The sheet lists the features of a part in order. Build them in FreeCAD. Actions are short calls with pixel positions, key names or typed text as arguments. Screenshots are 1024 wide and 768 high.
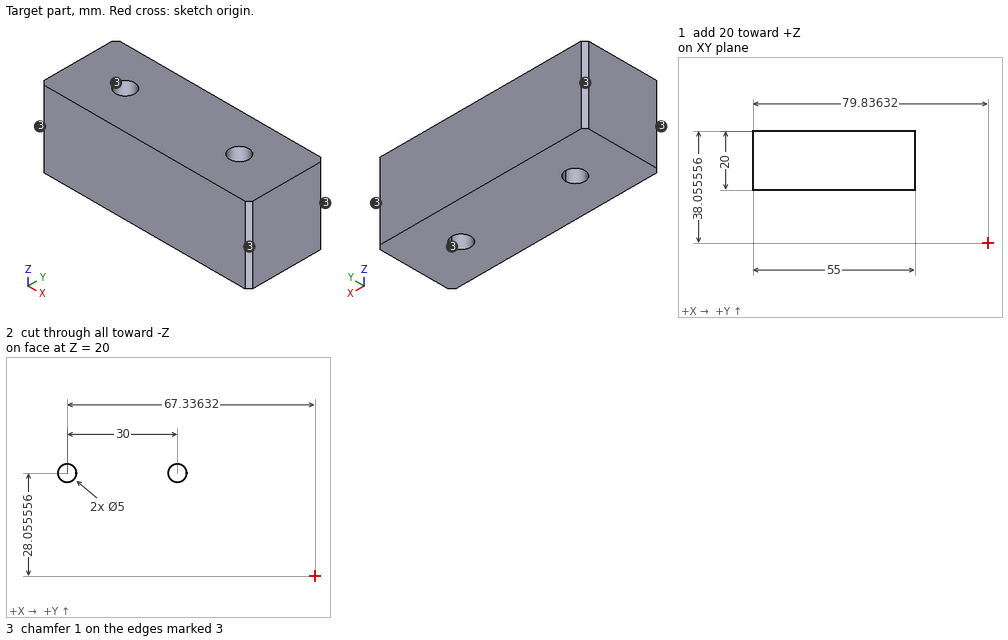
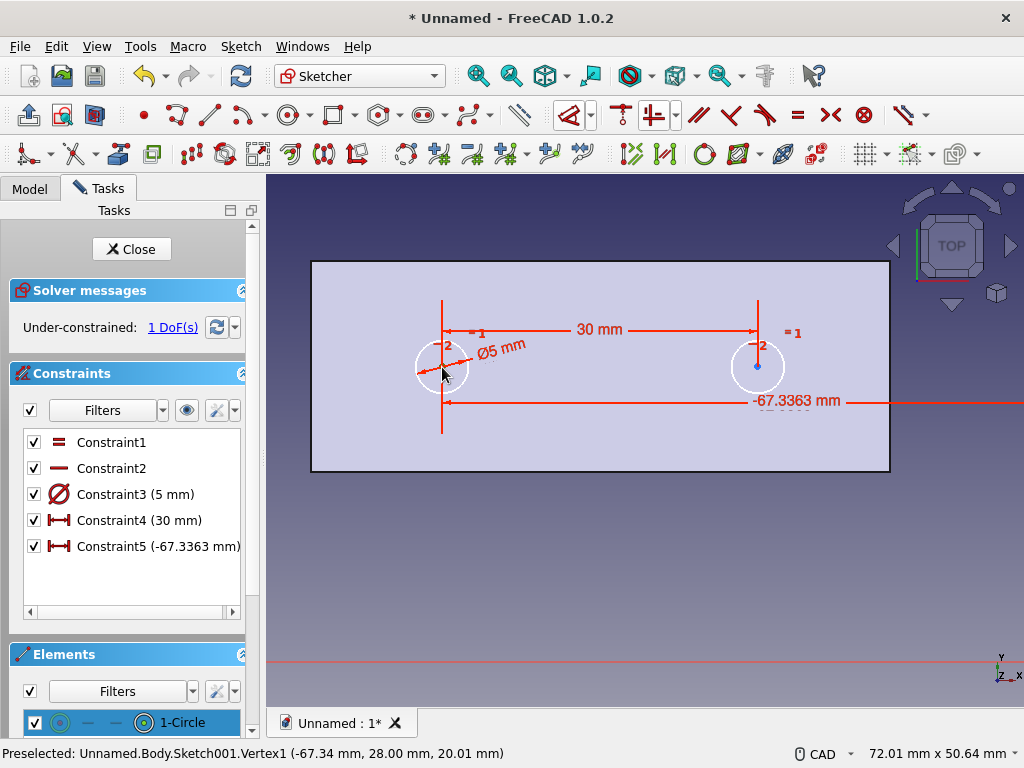
key(i)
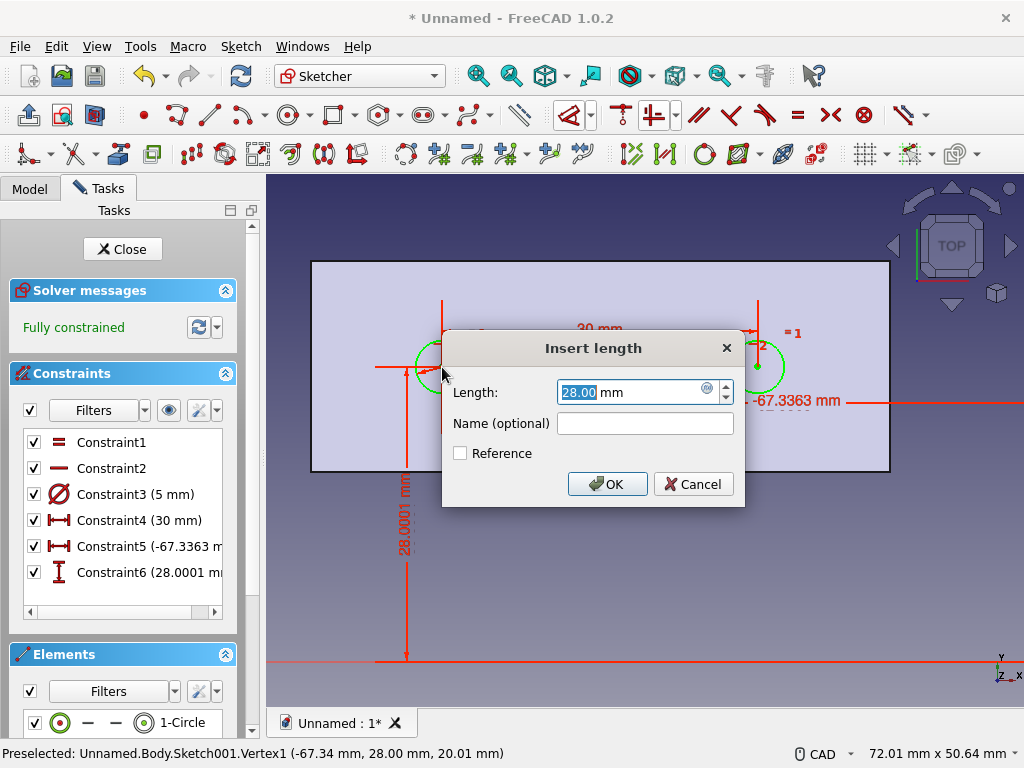
text(28.055556)
key(Return)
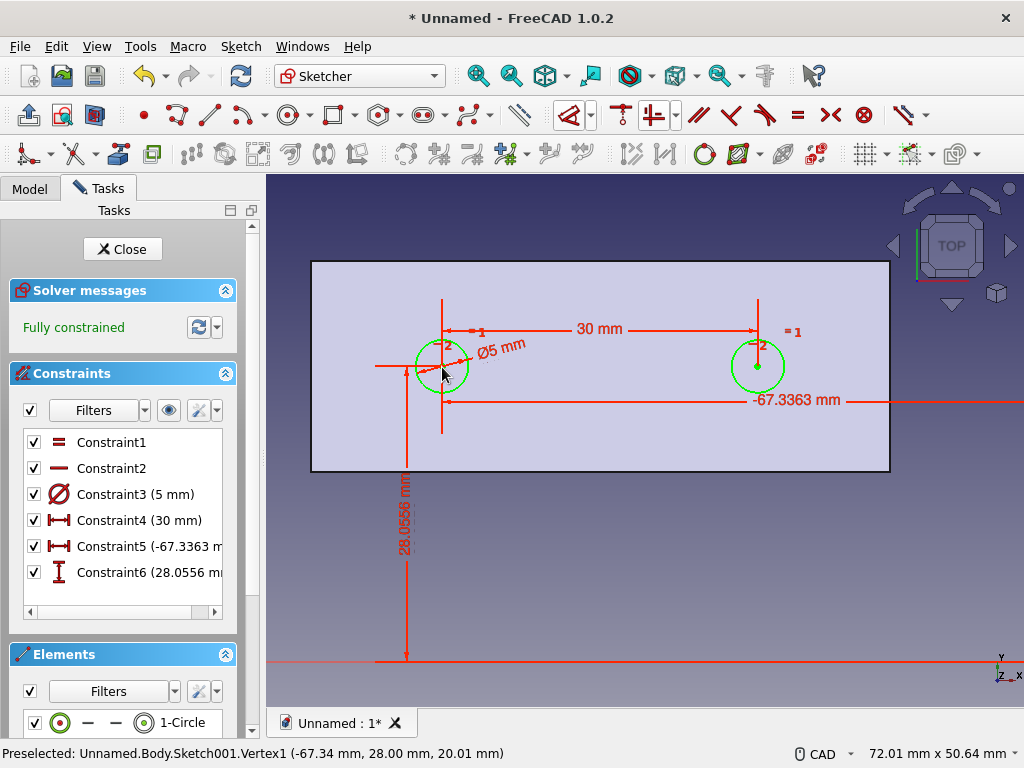
click(123, 249)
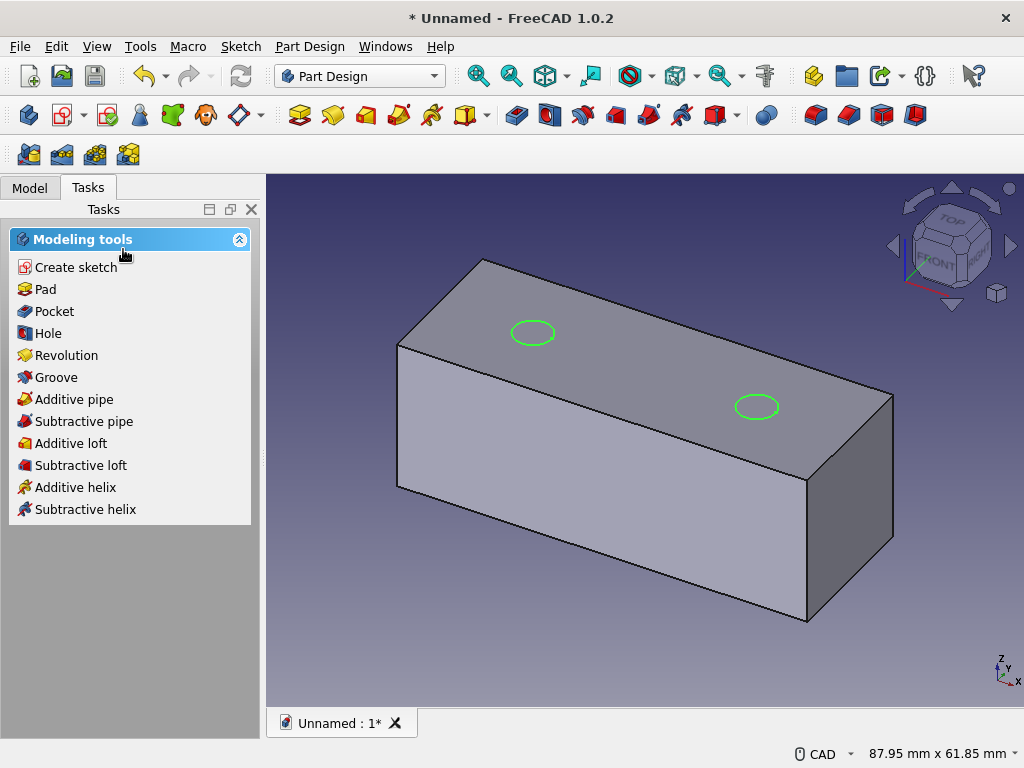
click(517, 116)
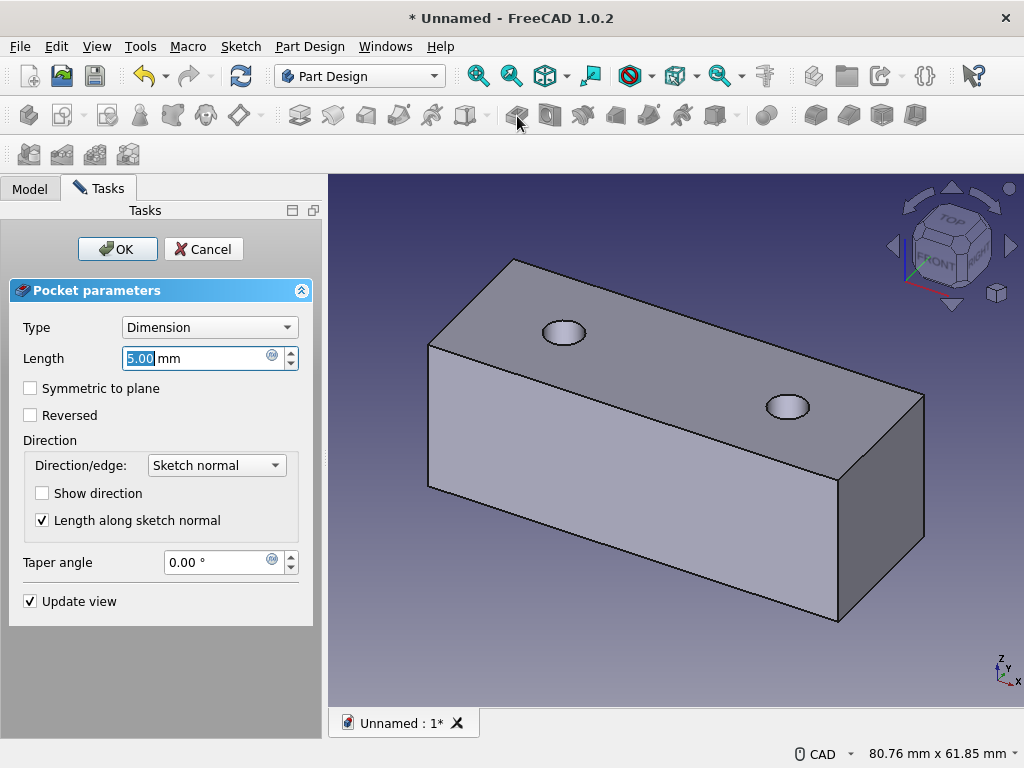
click(210, 328)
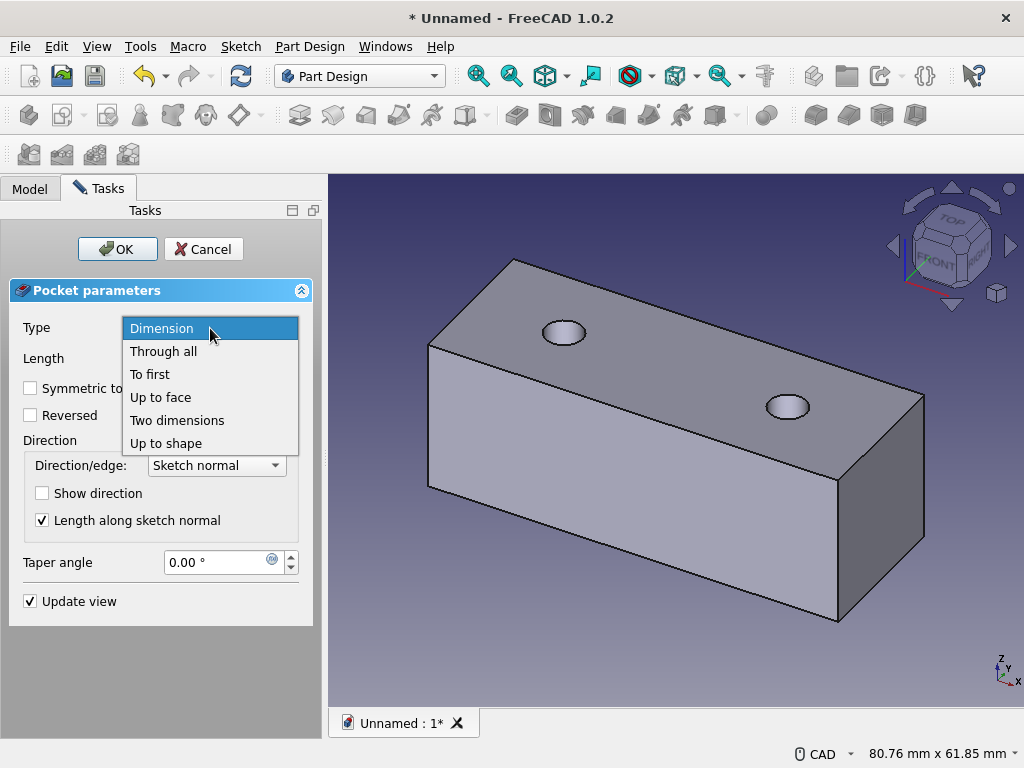
click(208, 352)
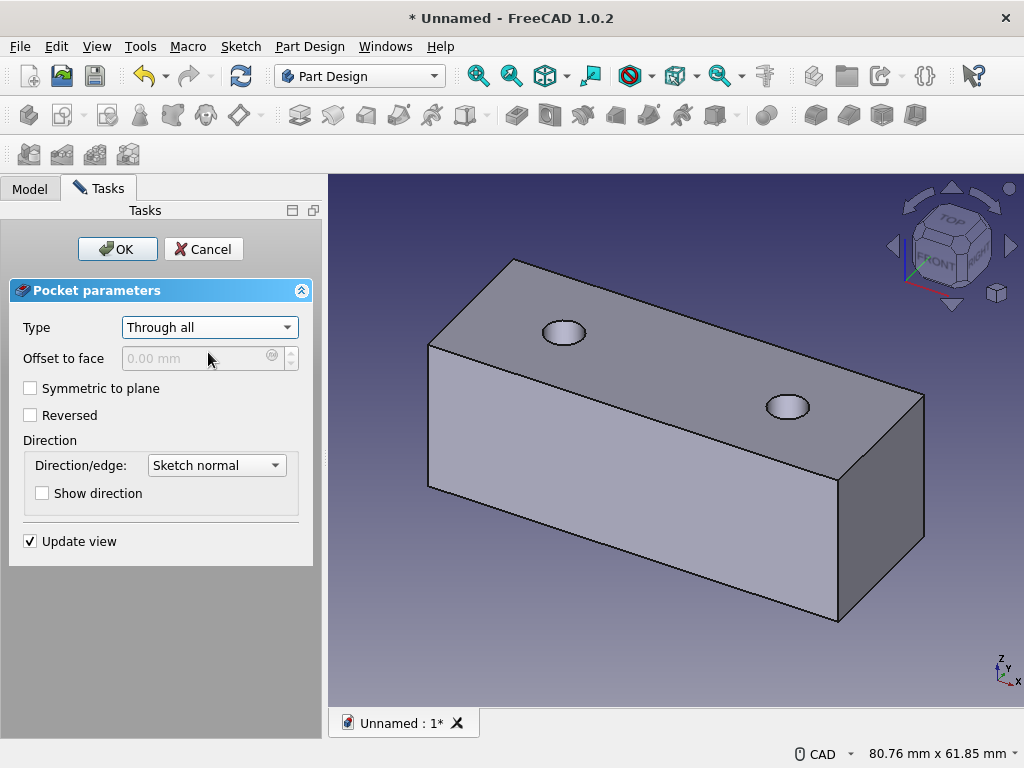
click(118, 249)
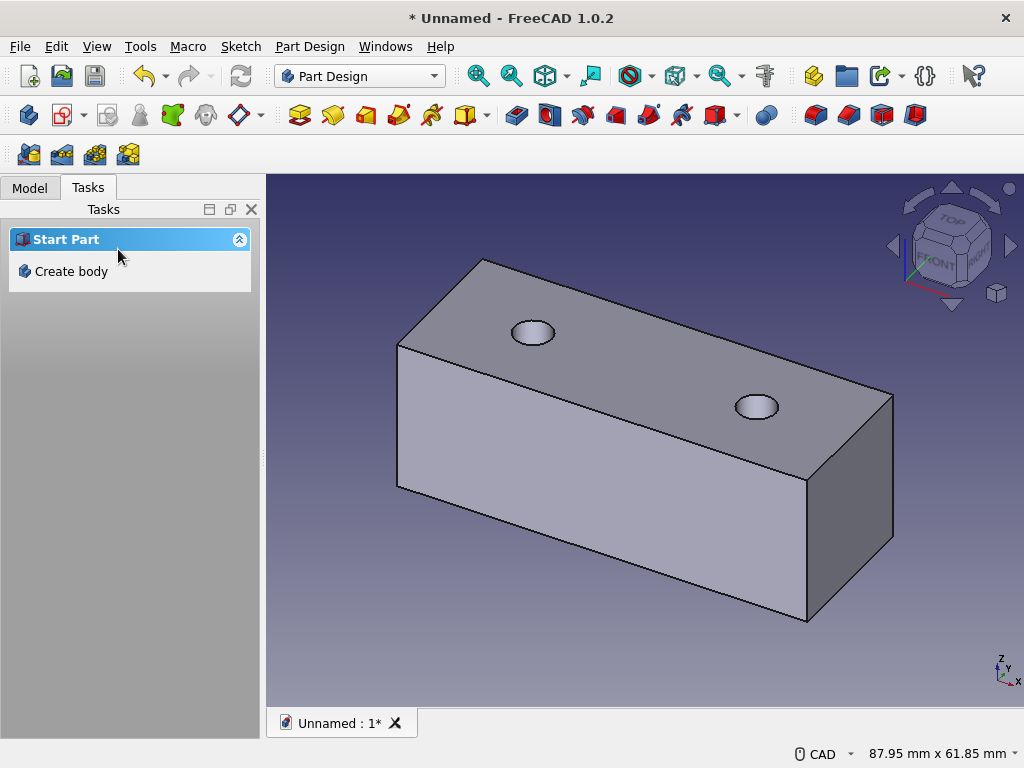
click(807, 550)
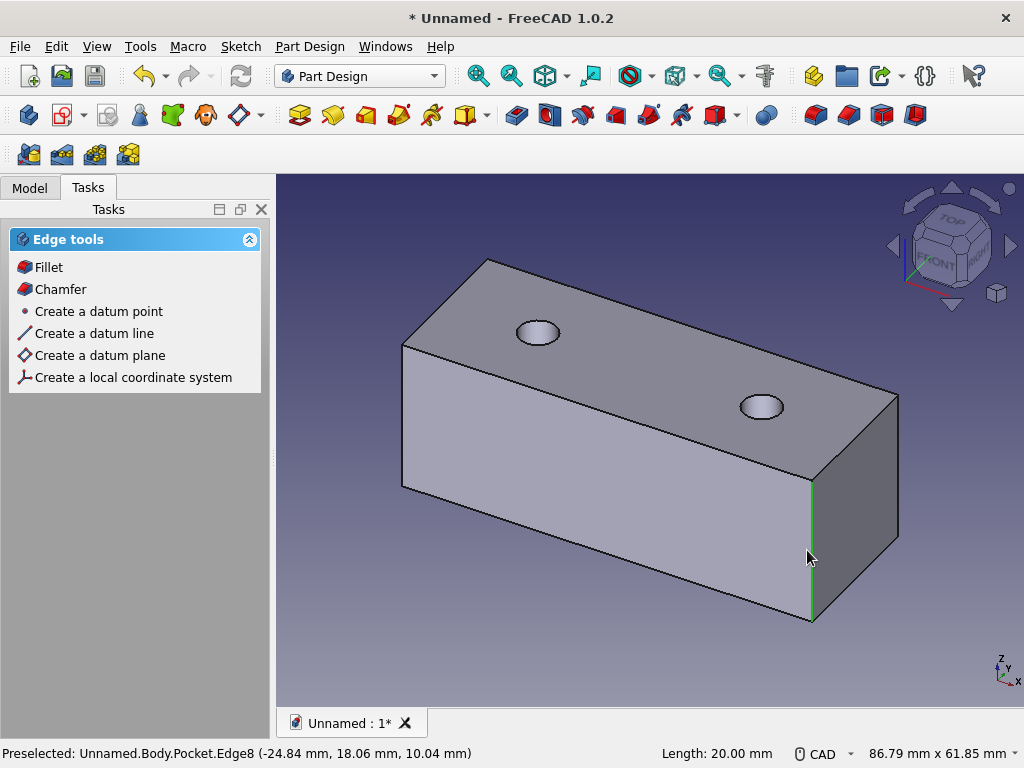
key(0)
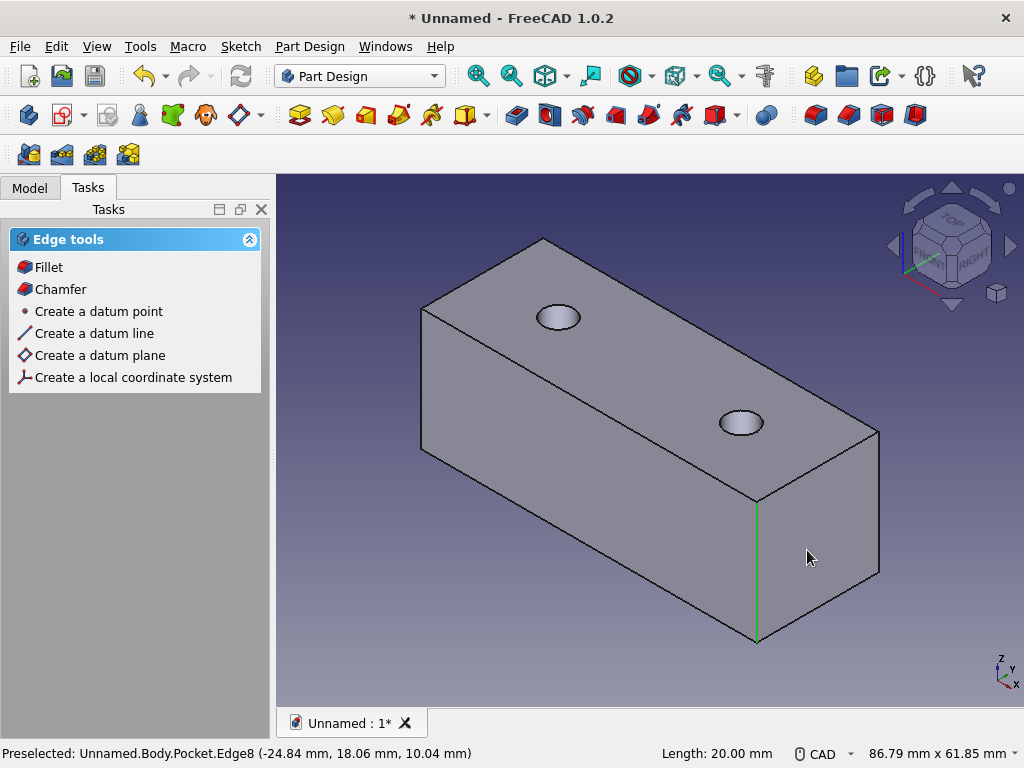
key(2)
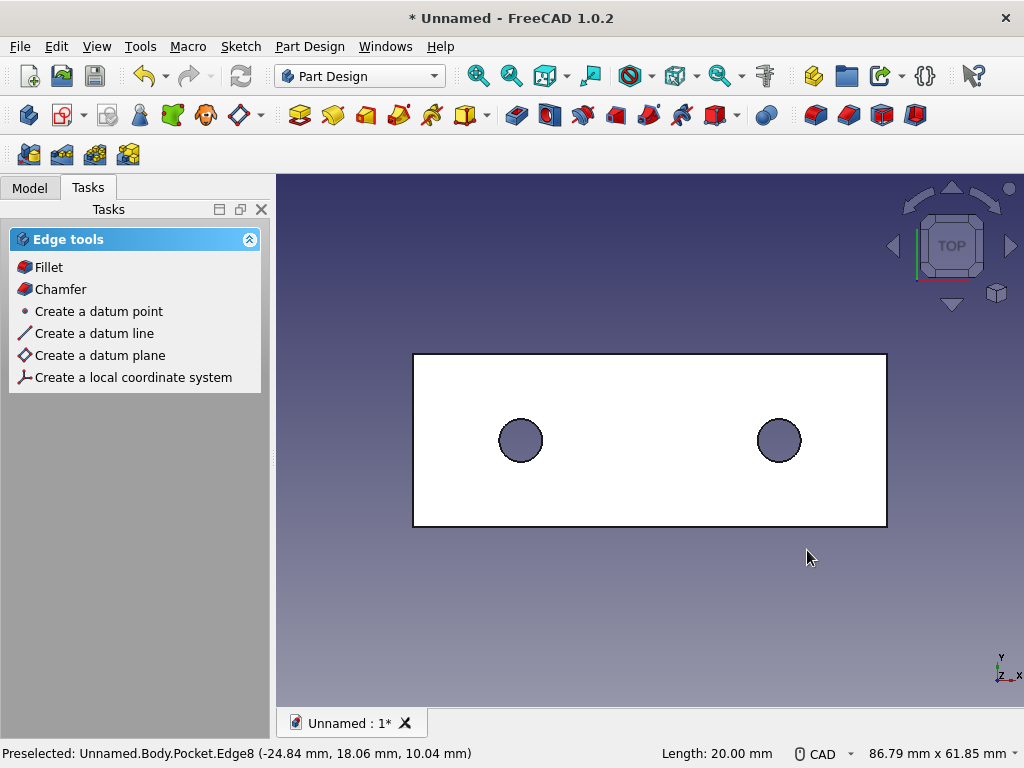
key(1)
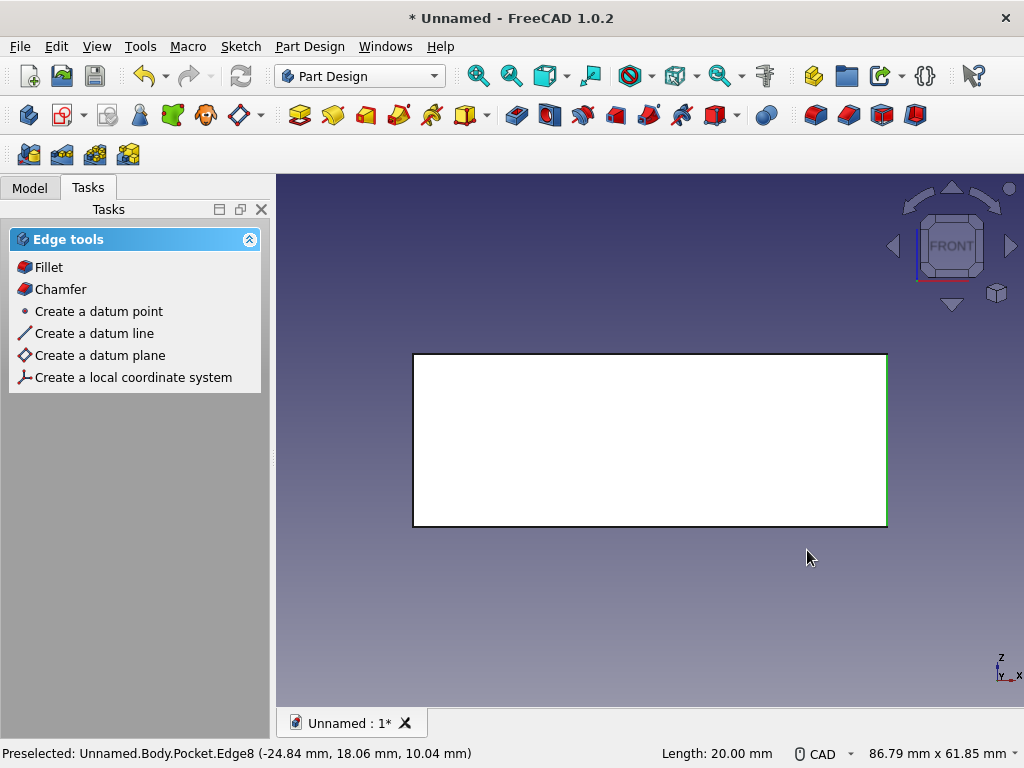
click(413, 440, ctrl)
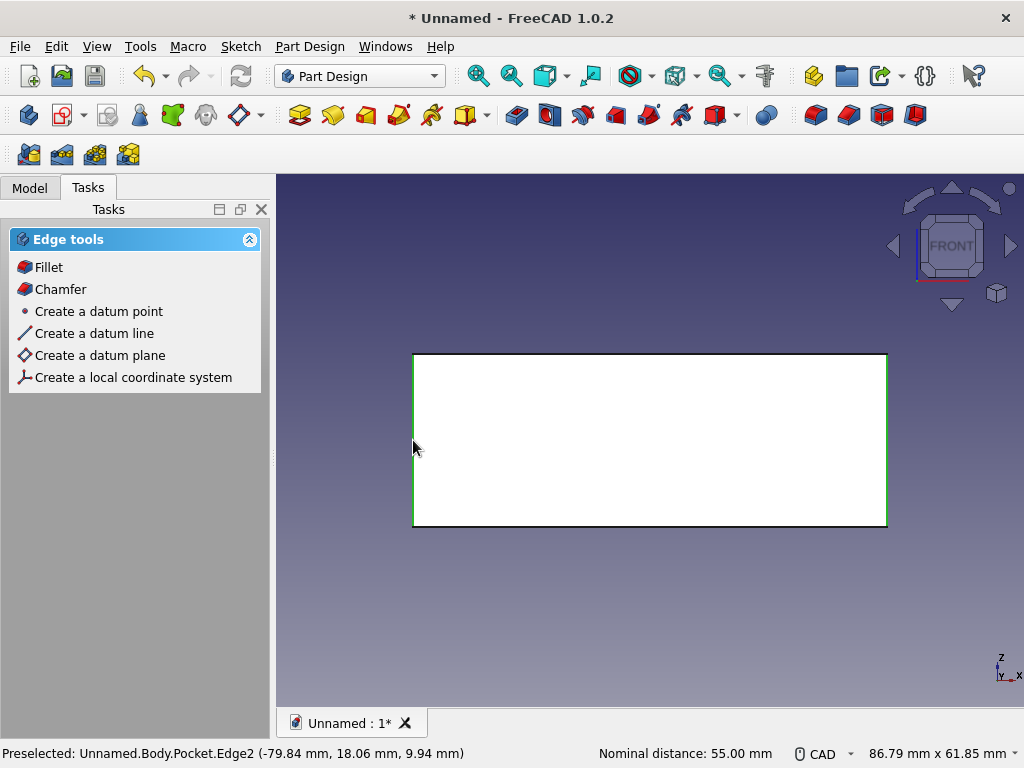
key(3)